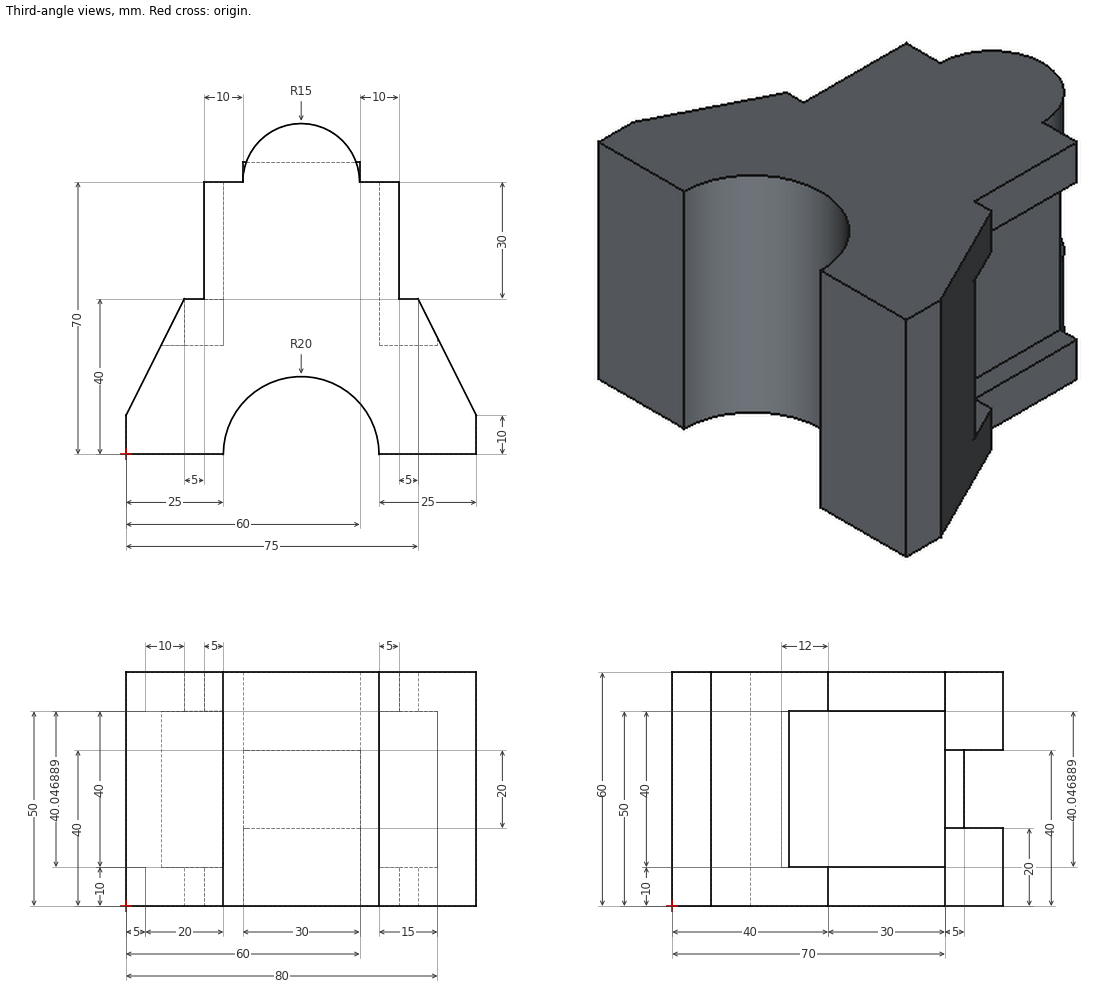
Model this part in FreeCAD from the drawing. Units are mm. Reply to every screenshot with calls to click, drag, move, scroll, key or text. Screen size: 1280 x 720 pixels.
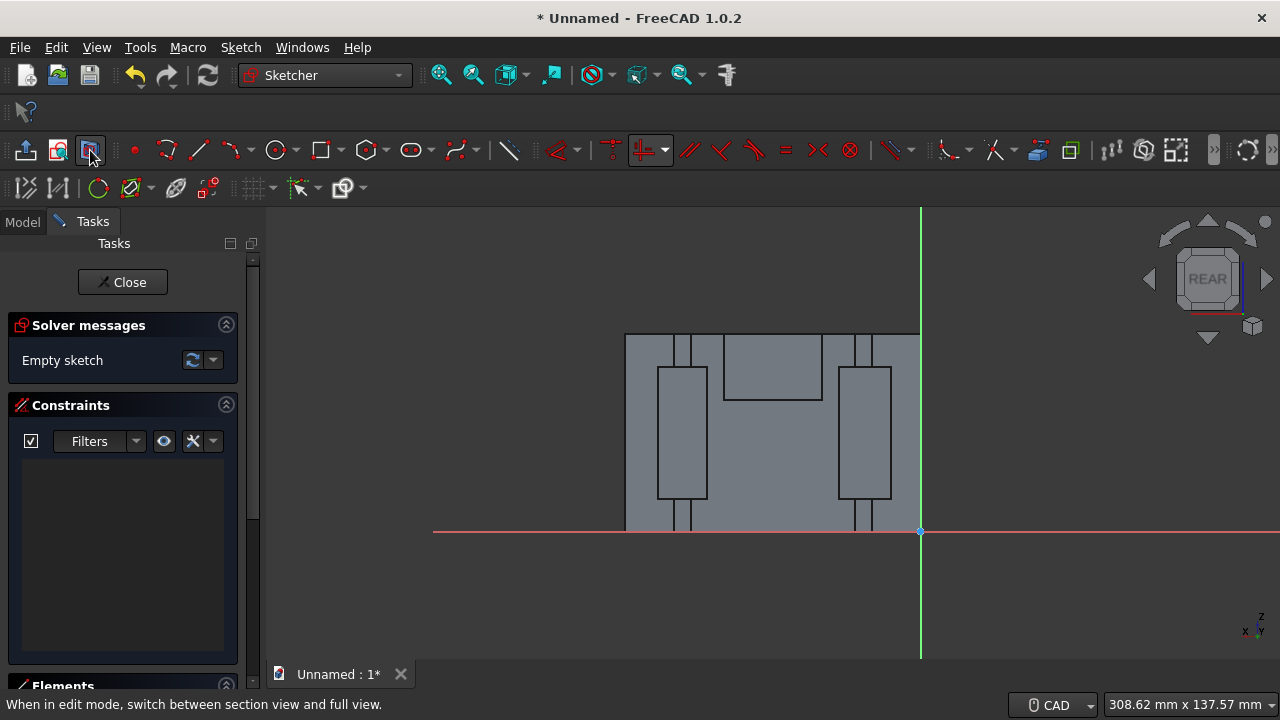
scroll(918, 493, up, 4)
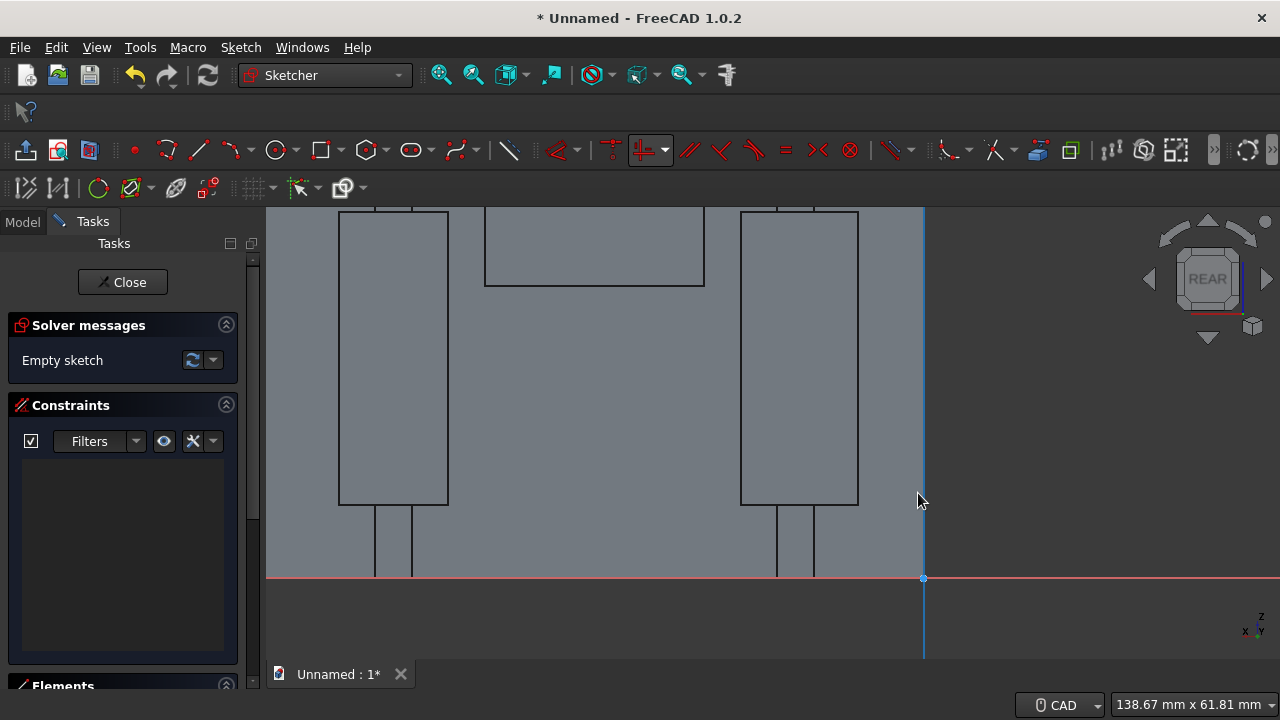
click(322, 150)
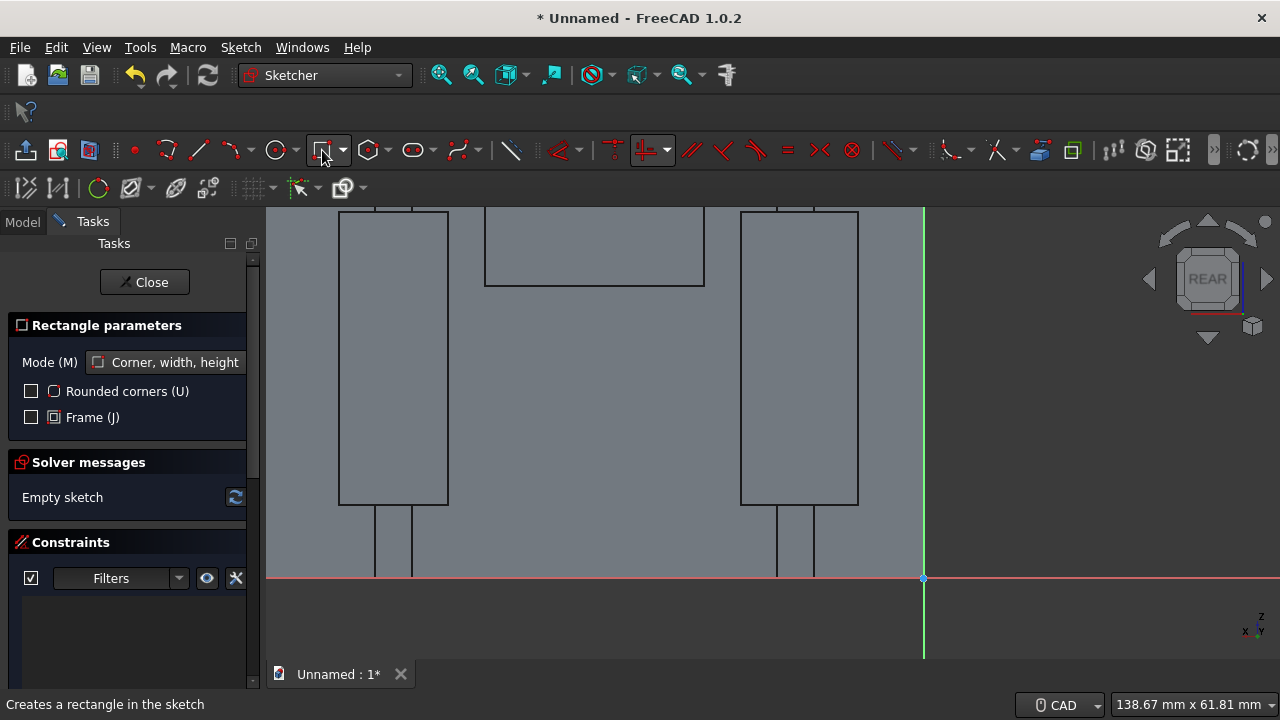
click(485, 286)
click(704, 432)
key(Escape)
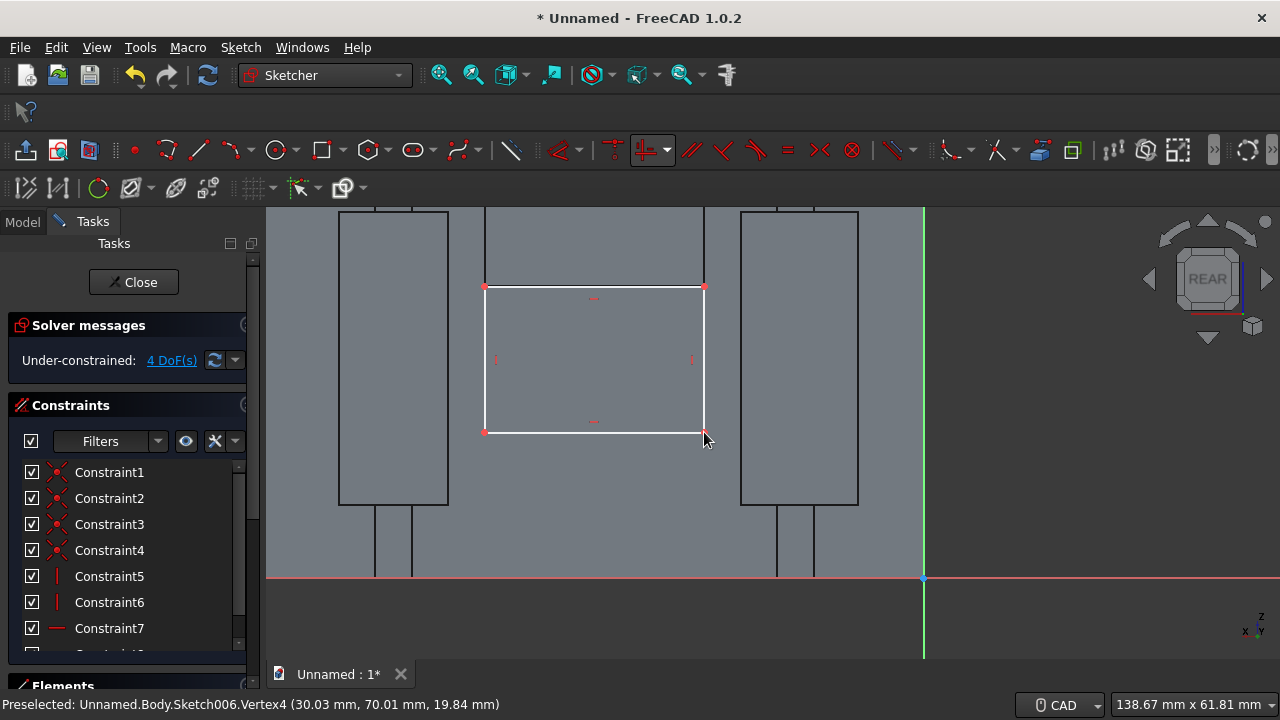
click(558, 150)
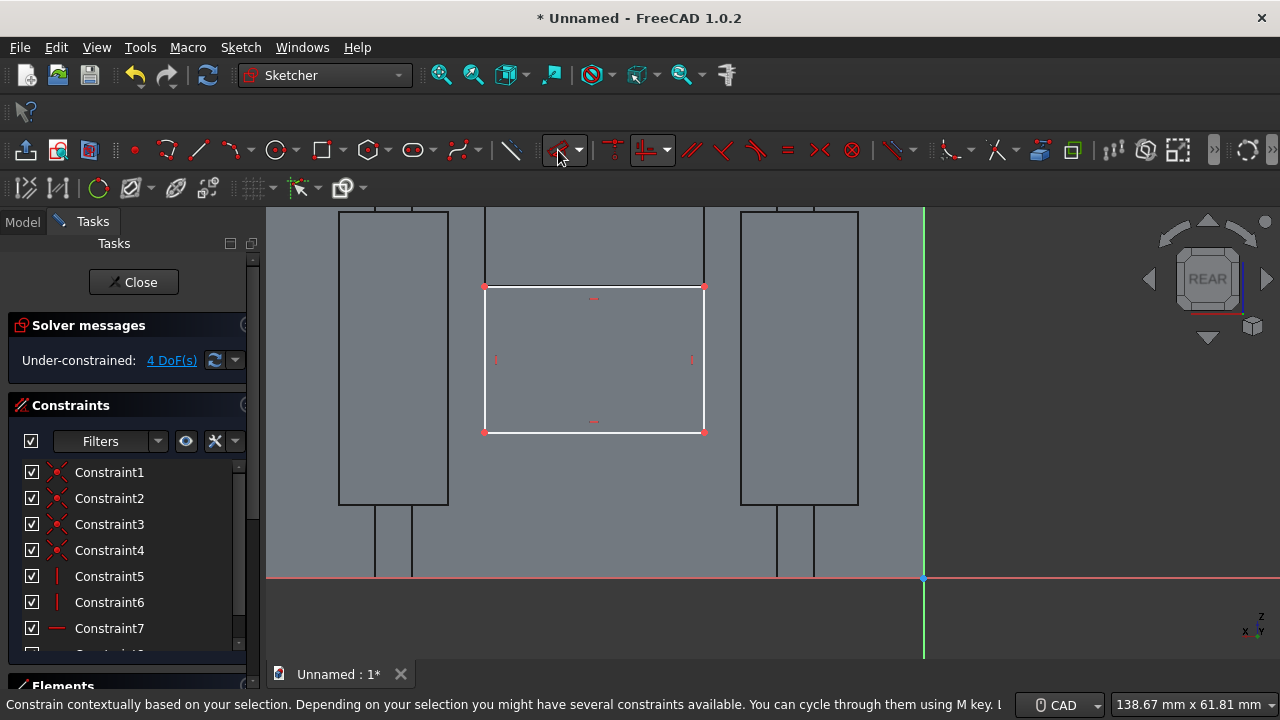
click(485, 331)
click(451, 360)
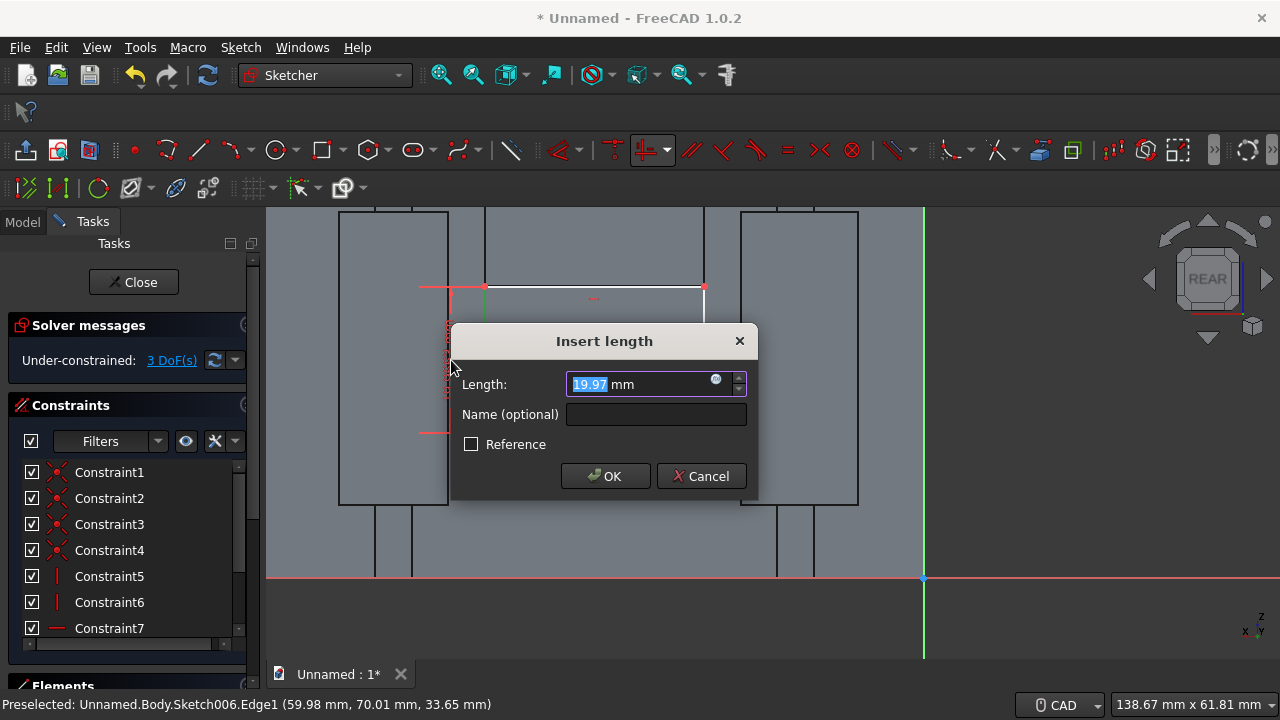
text(20)
key(Return)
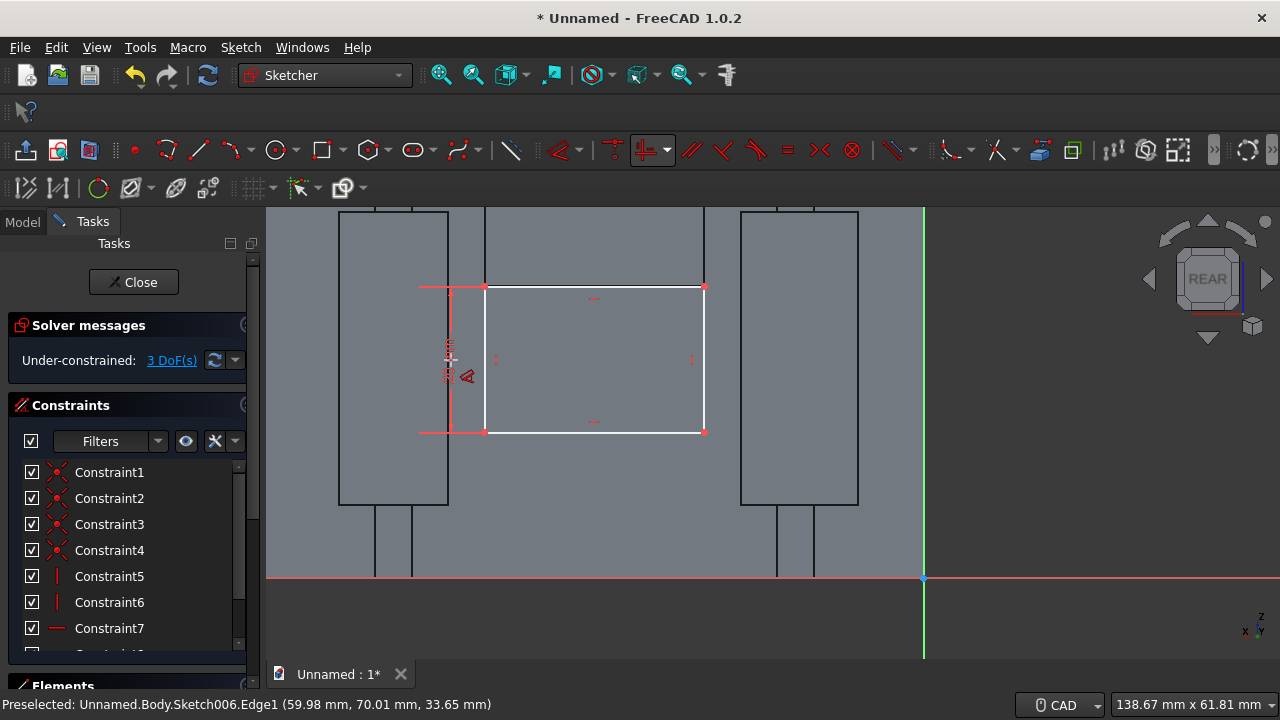
click(551, 433)
click(594, 467)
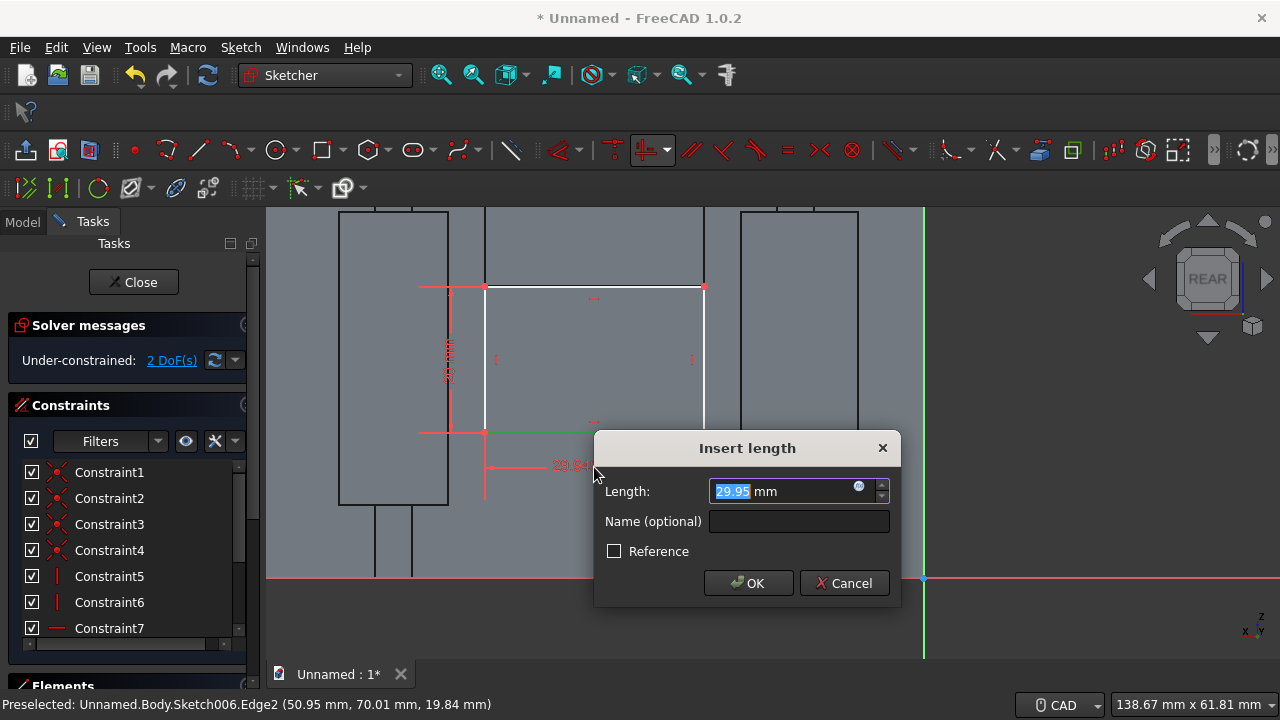
text(30)
key(Return)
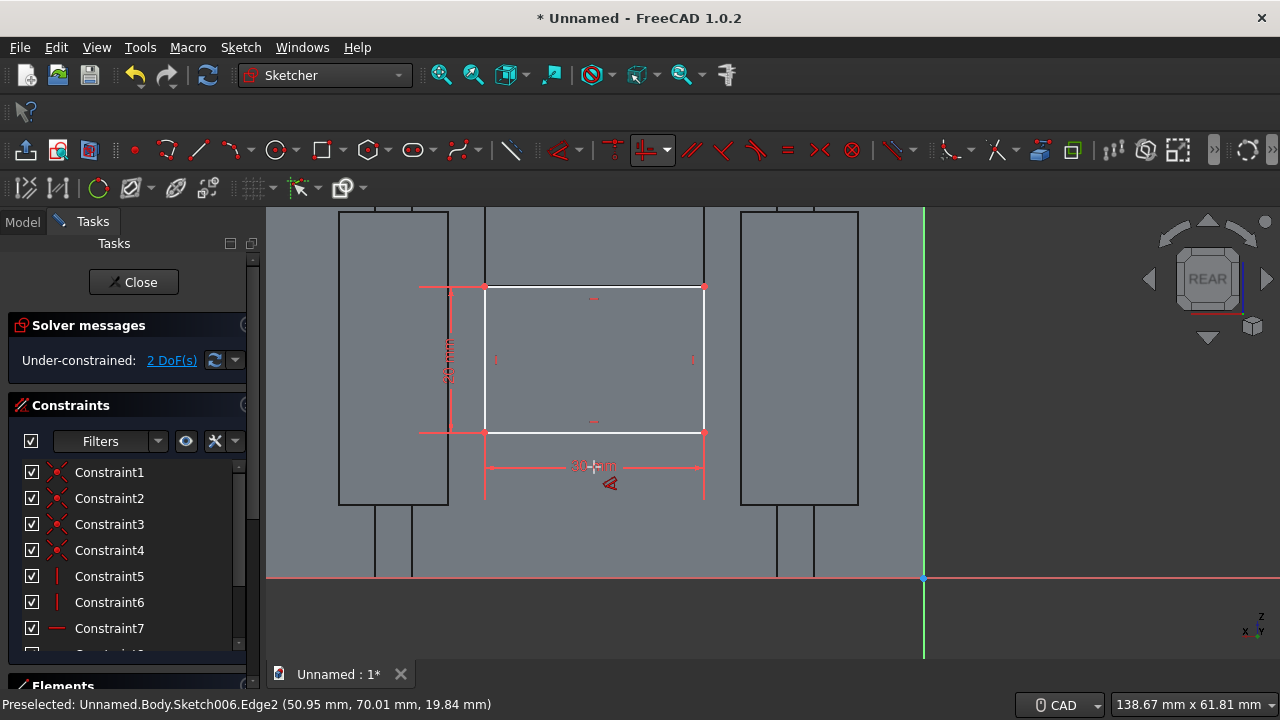
click(485, 287)
click(704, 612)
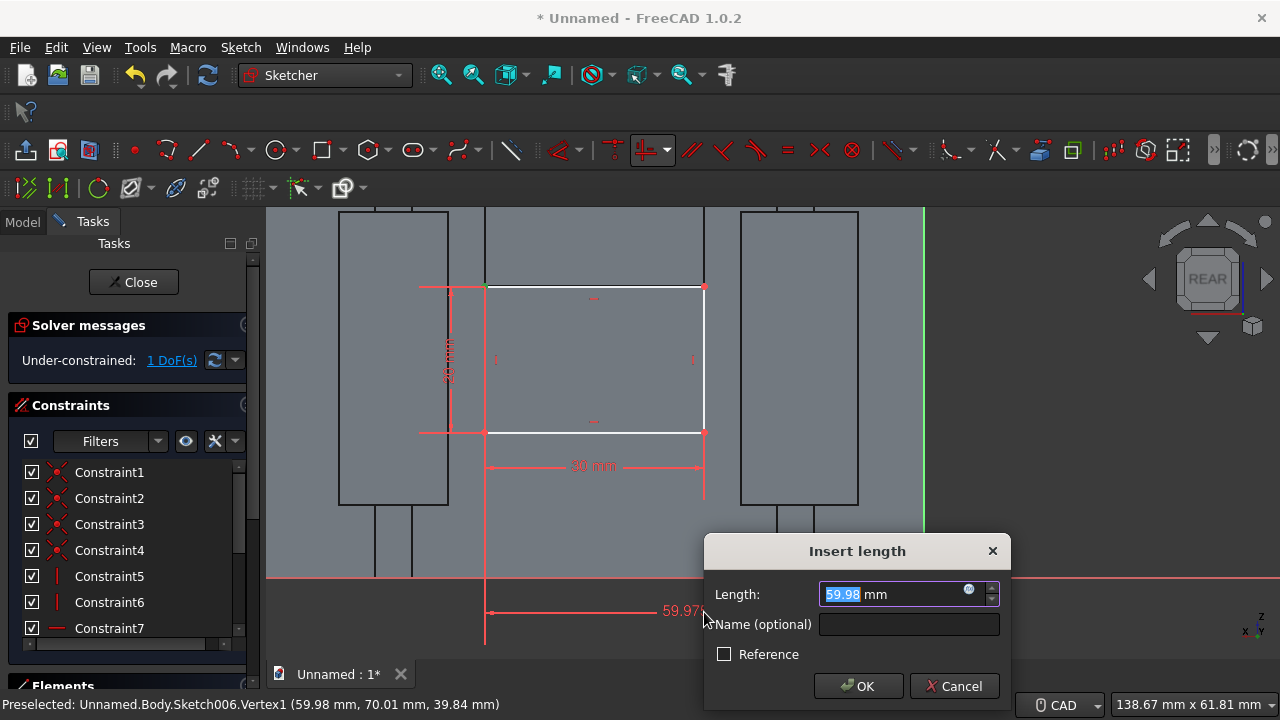
text(60)
key(Return)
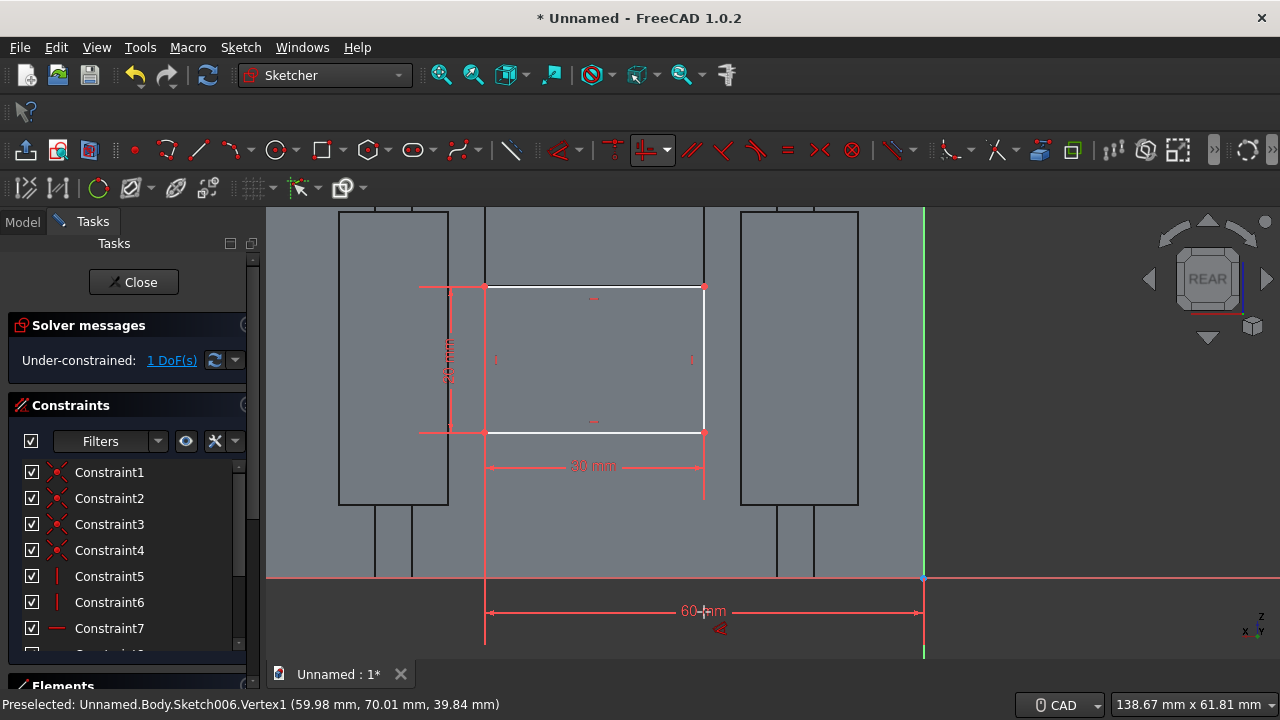
click(485, 287)
click(958, 432)